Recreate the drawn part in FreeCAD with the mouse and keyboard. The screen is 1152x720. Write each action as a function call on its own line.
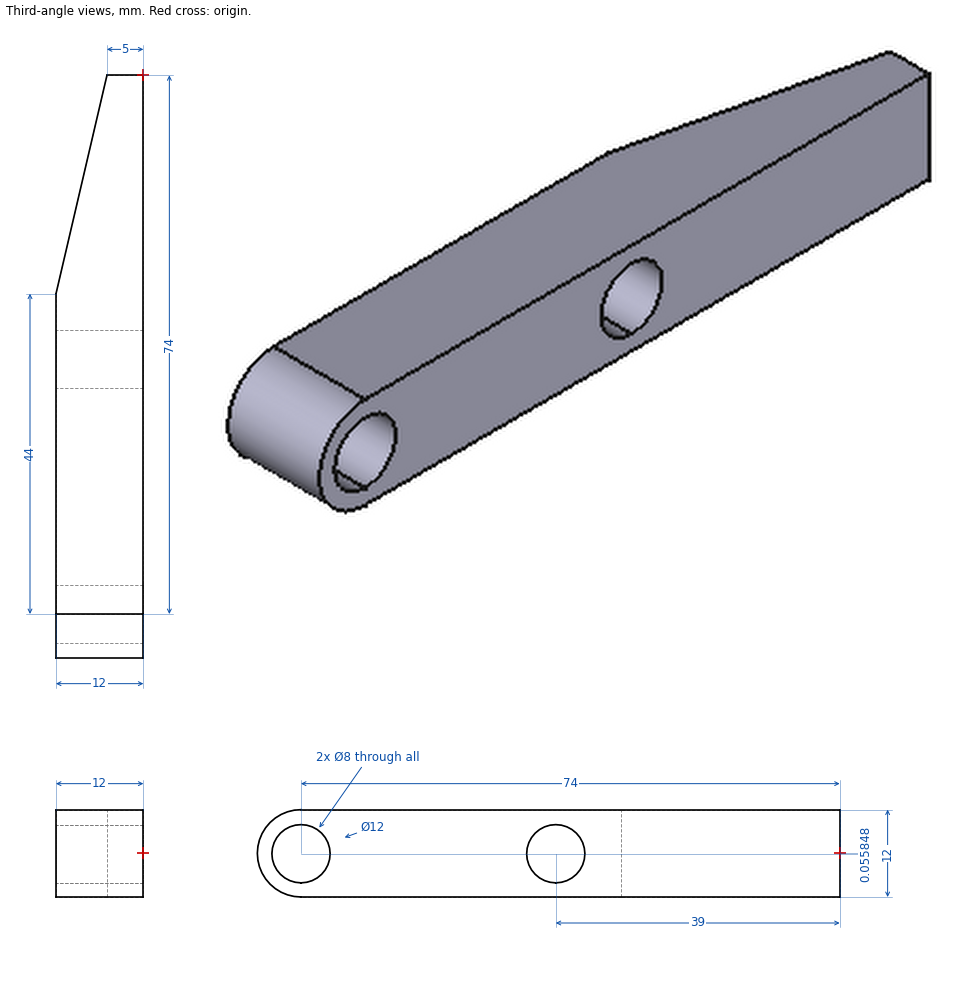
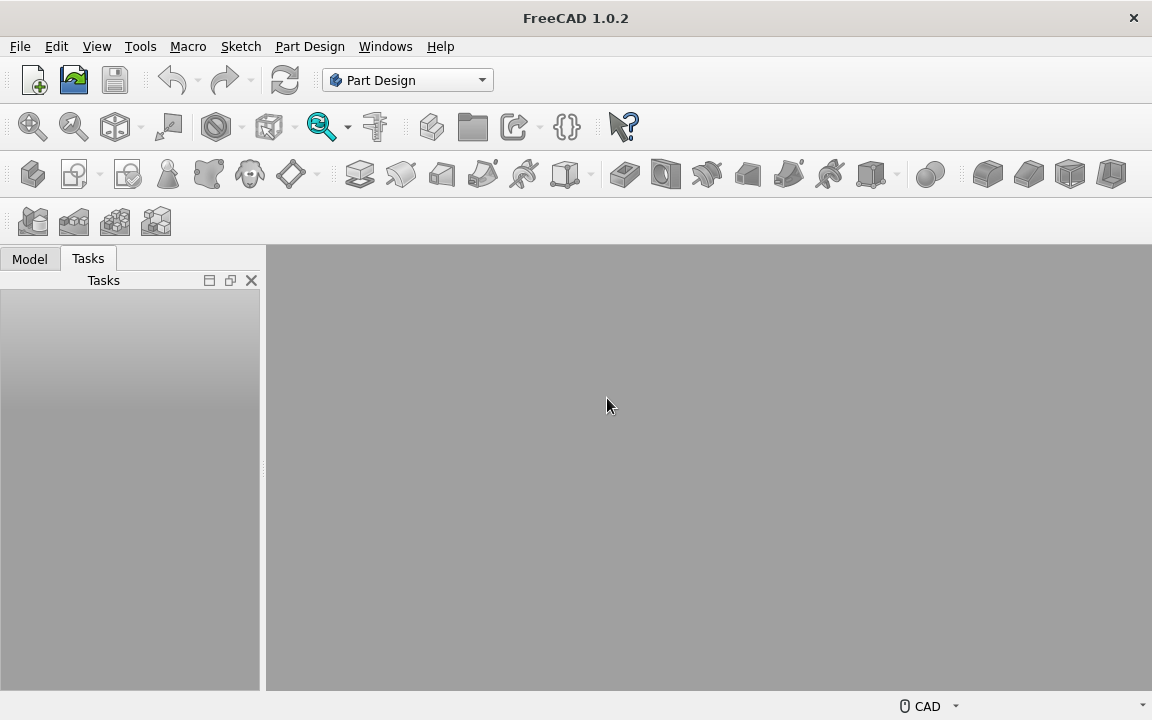
click(33, 80)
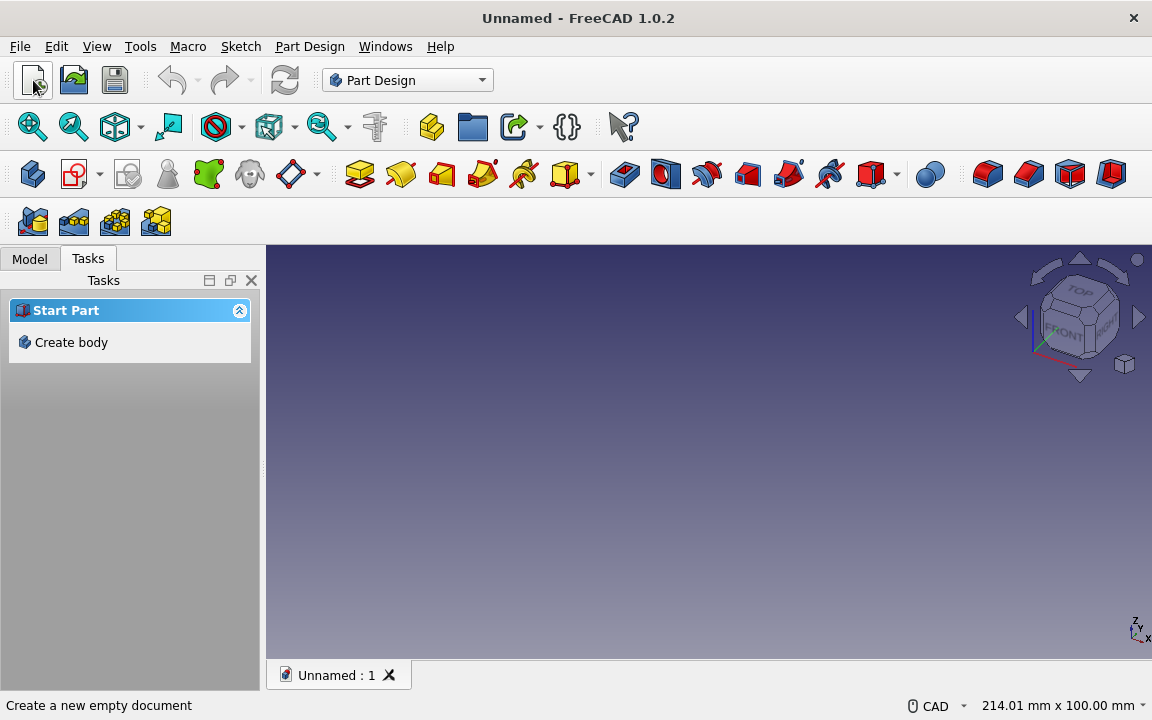
click(74, 174)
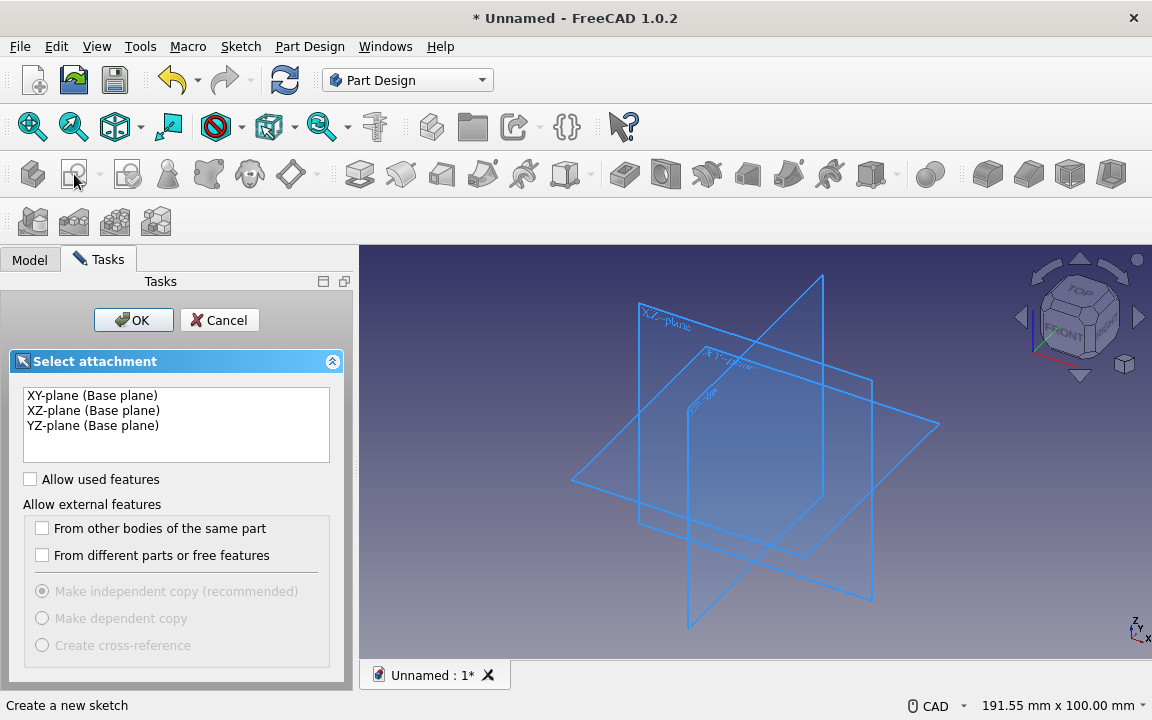
click(84, 396)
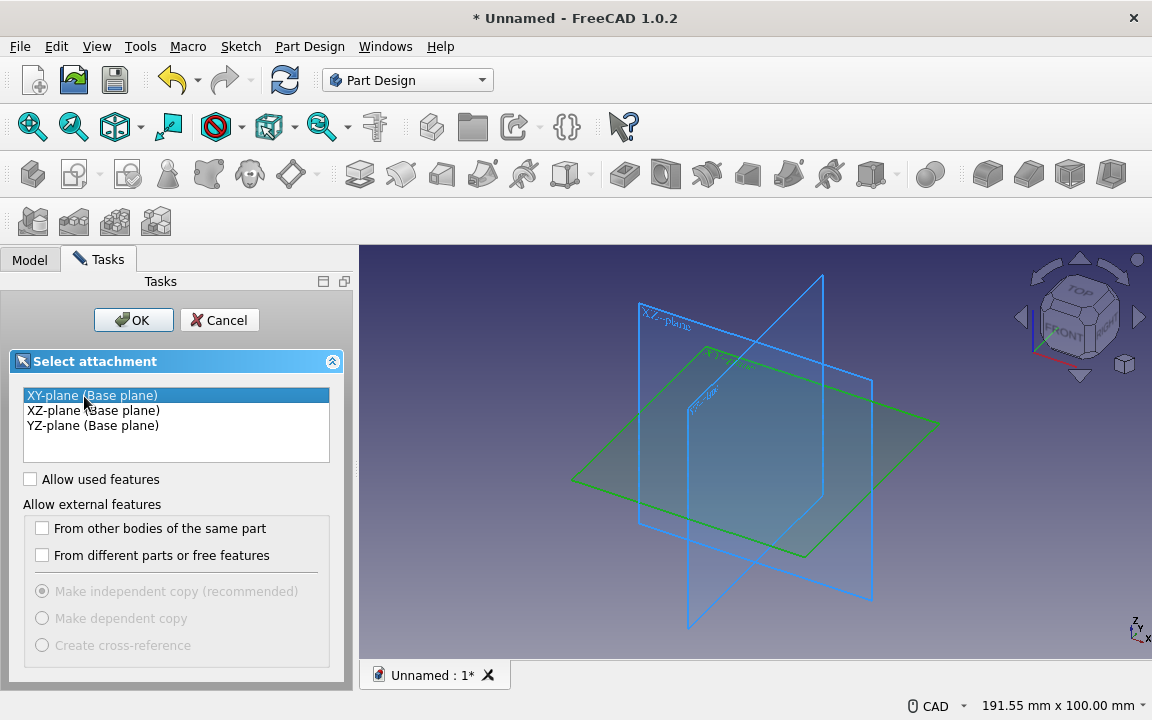
click(134, 320)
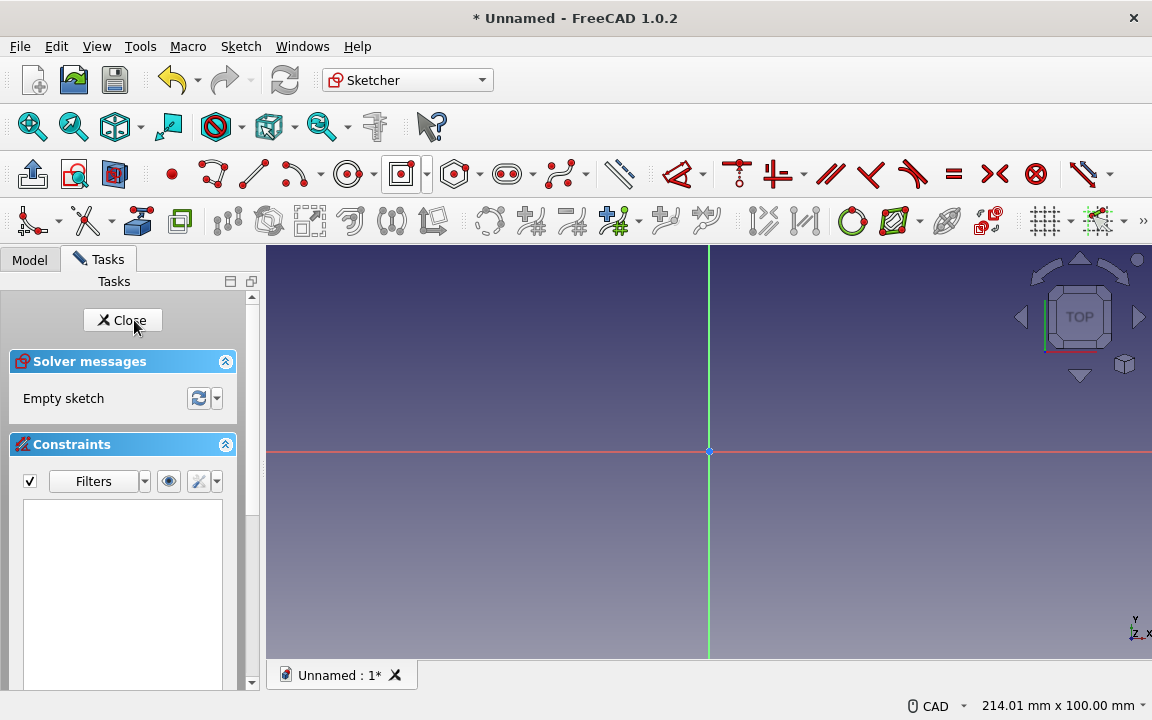
scroll(552, 273, down, 2)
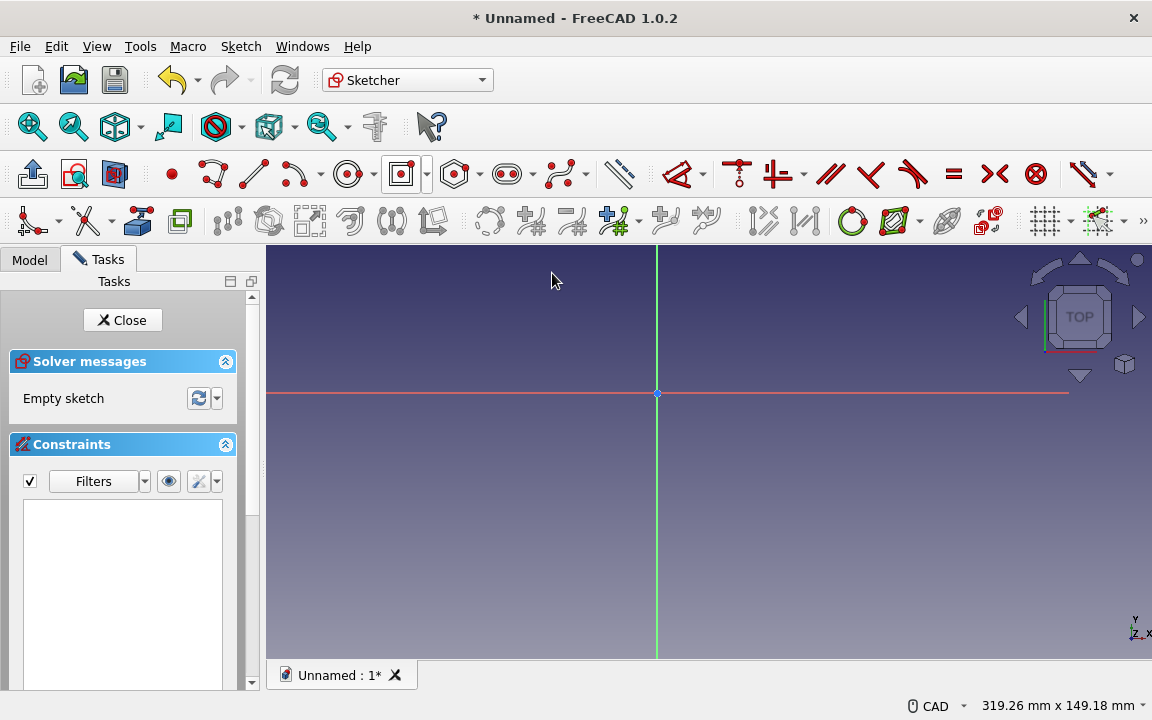
click(213, 174)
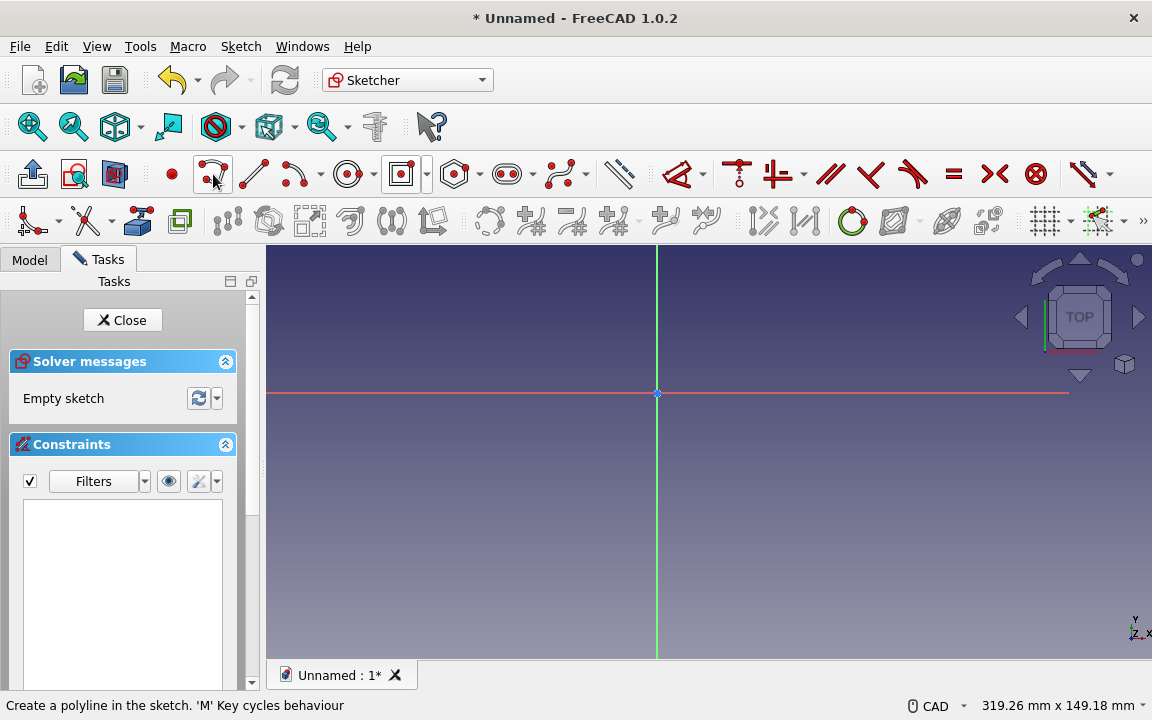
click(657, 393)
click(643, 402)
click(624, 476)
click(624, 598)
click(648, 598)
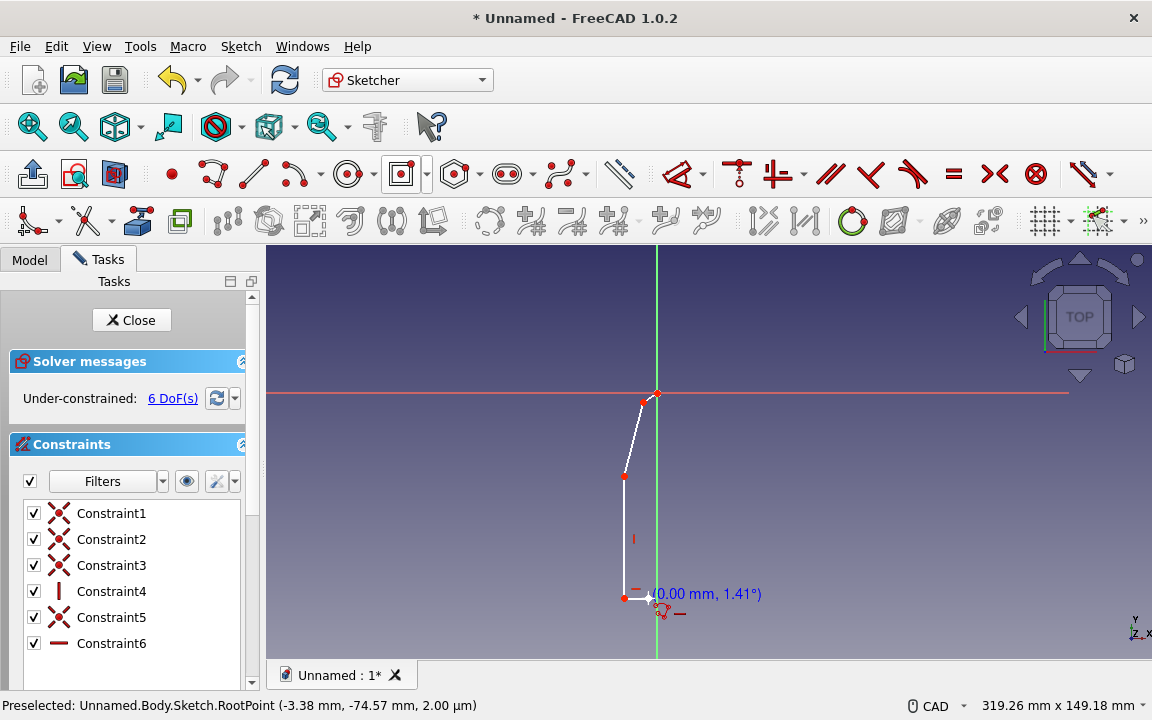
scroll(657, 393, up, 5)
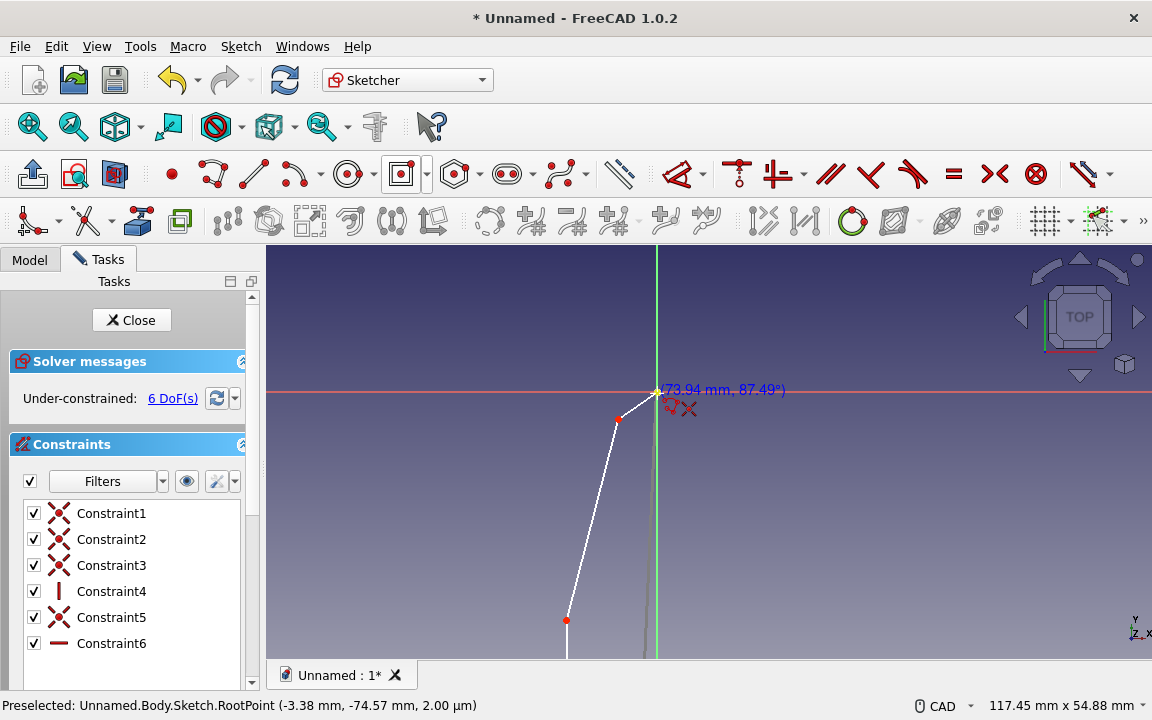
click(657, 392)
key(Escape)
key(Escape)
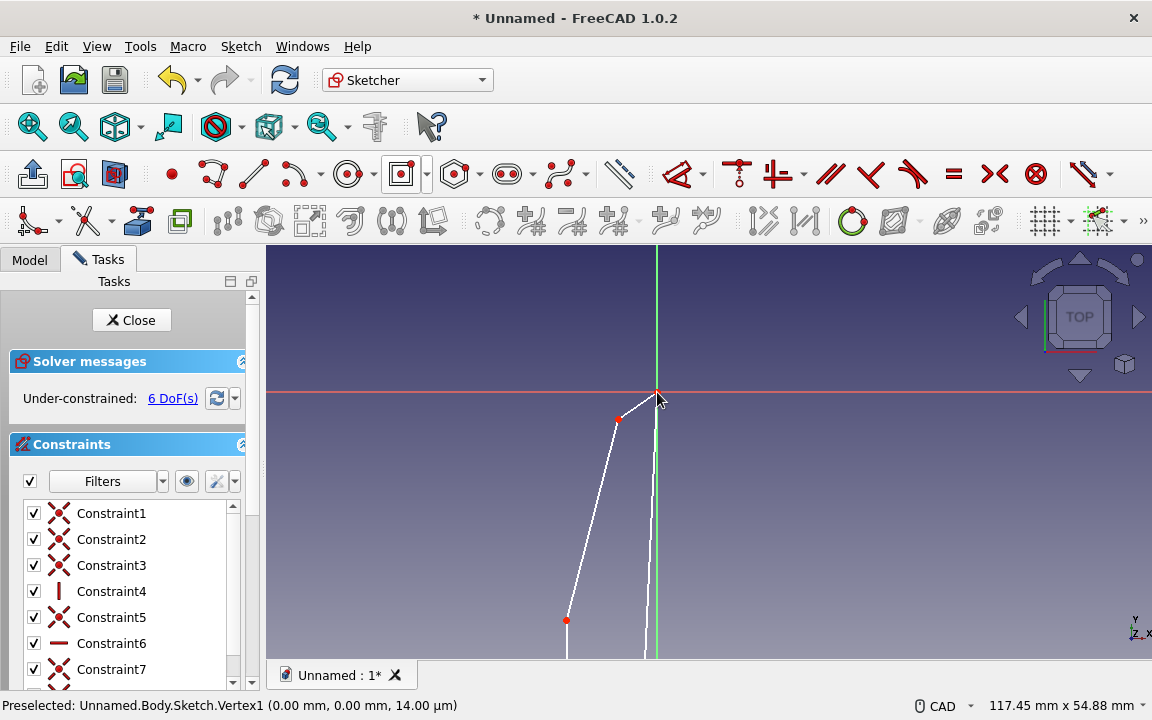
click(630, 411)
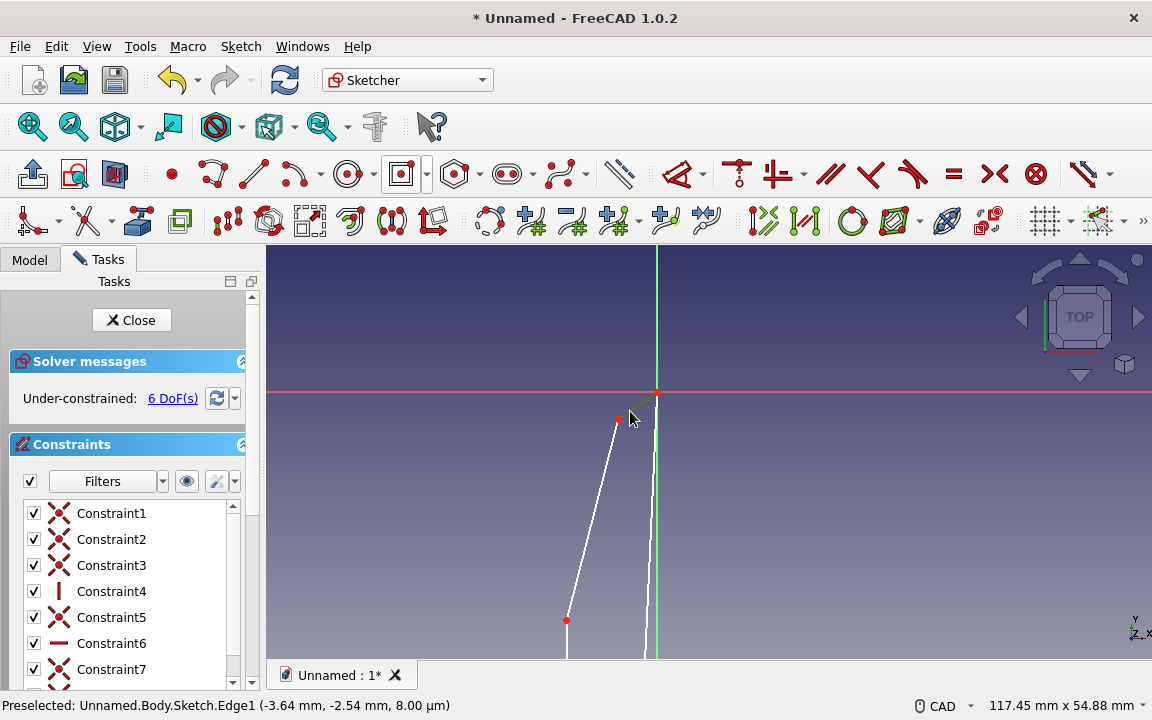
key(h)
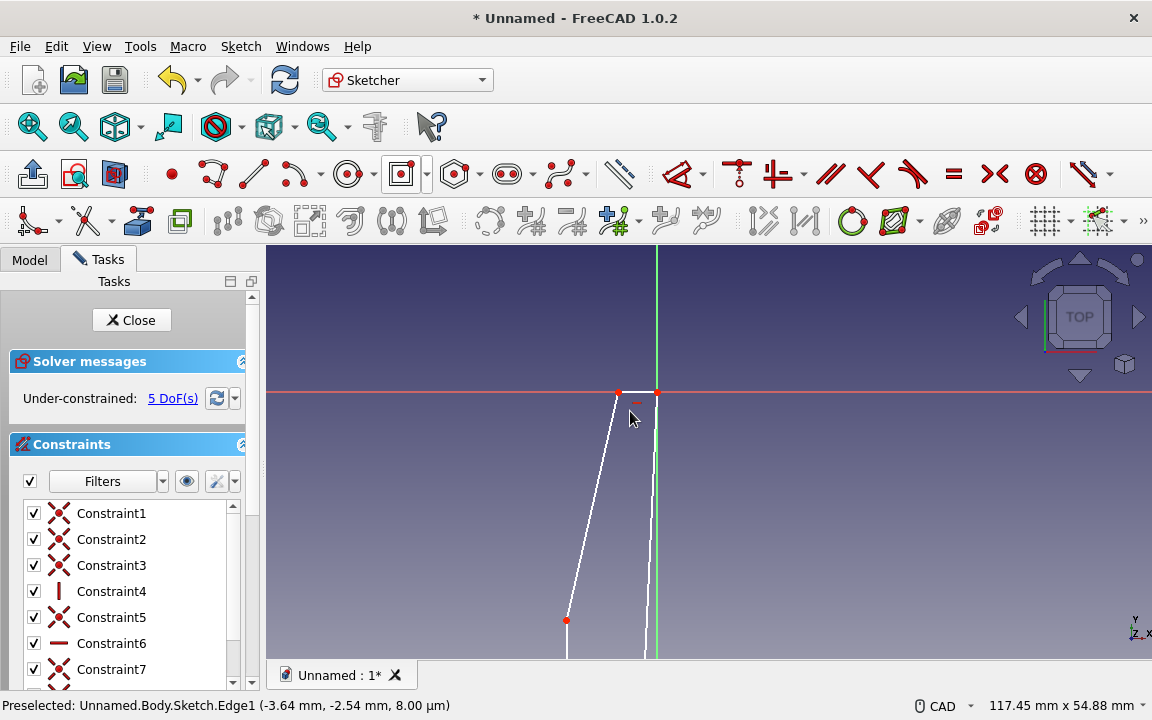
scroll(647, 616, up, 2)